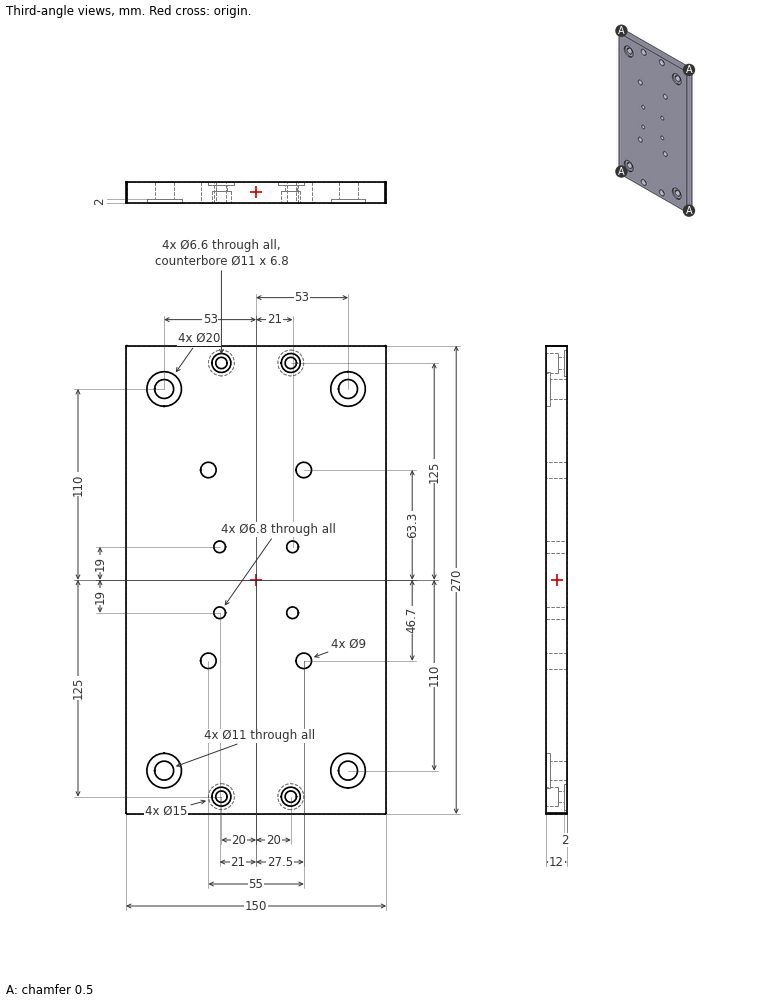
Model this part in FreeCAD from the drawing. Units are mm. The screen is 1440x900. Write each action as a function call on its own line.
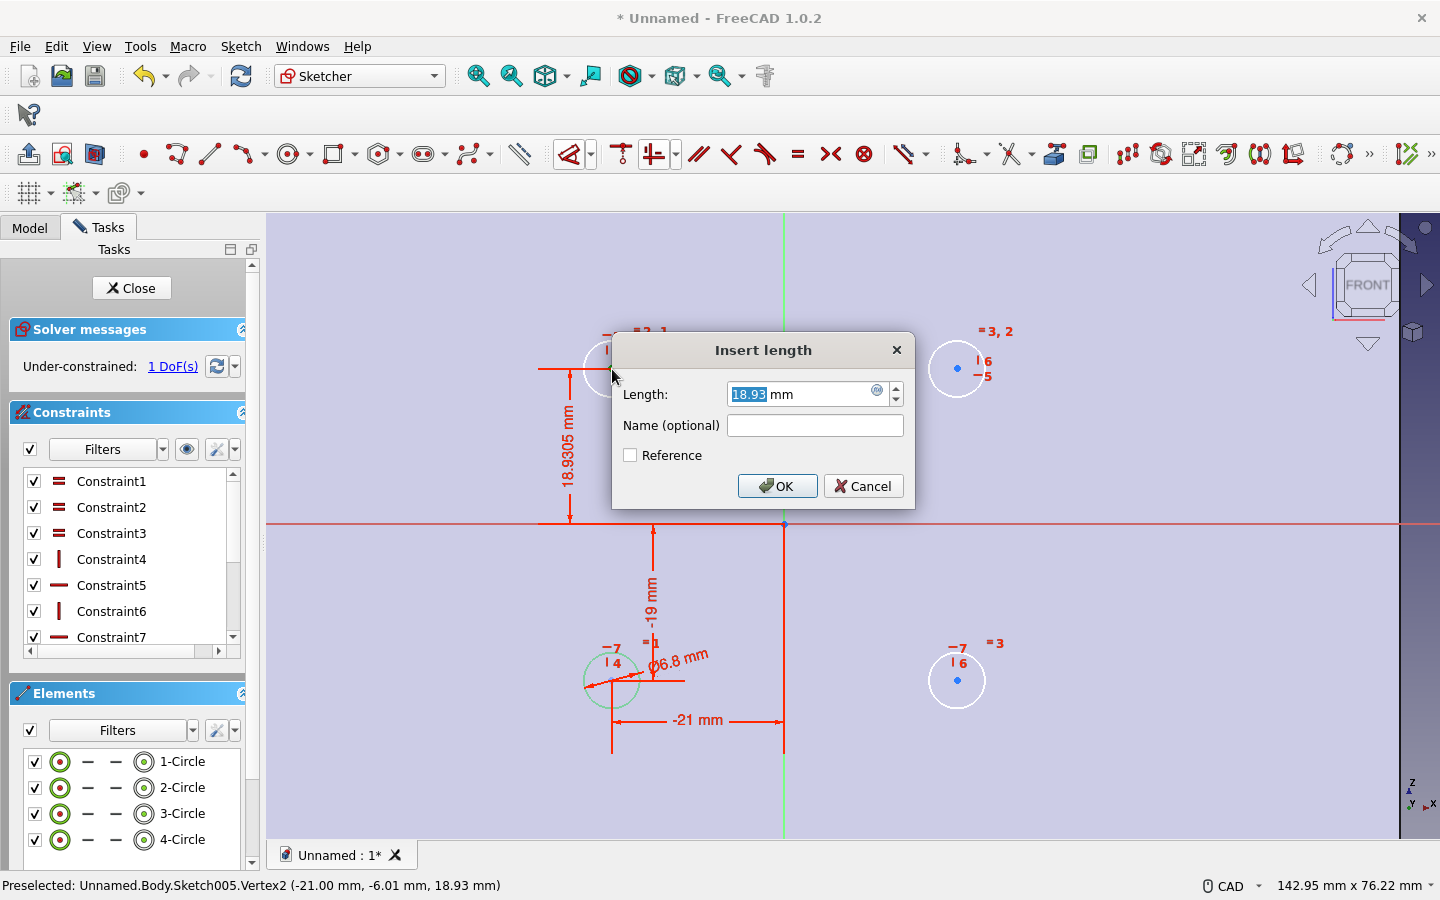
text(19)
key(Return)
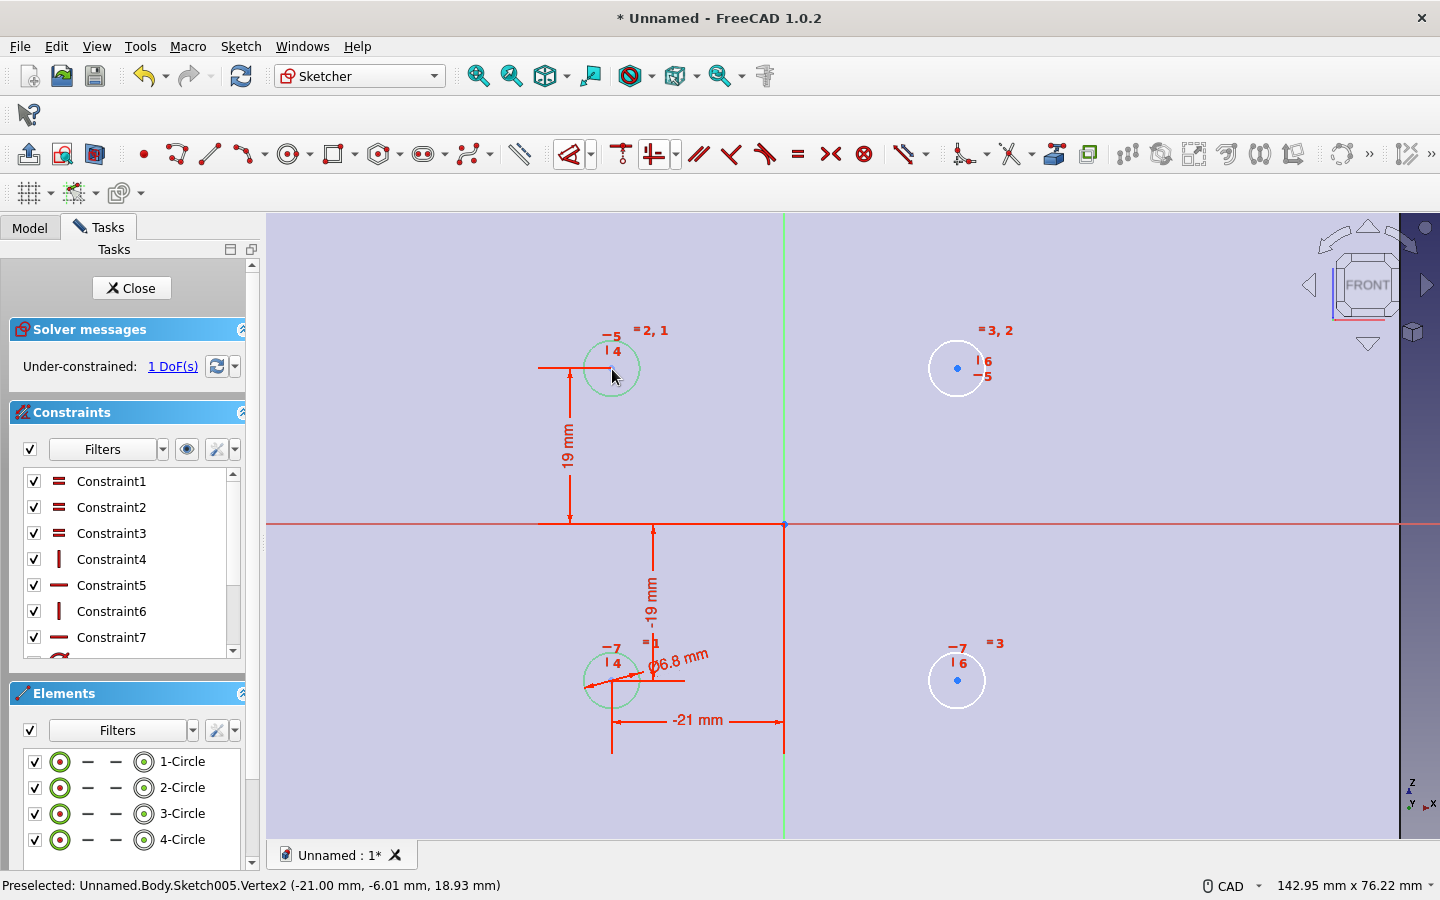
click(957, 368)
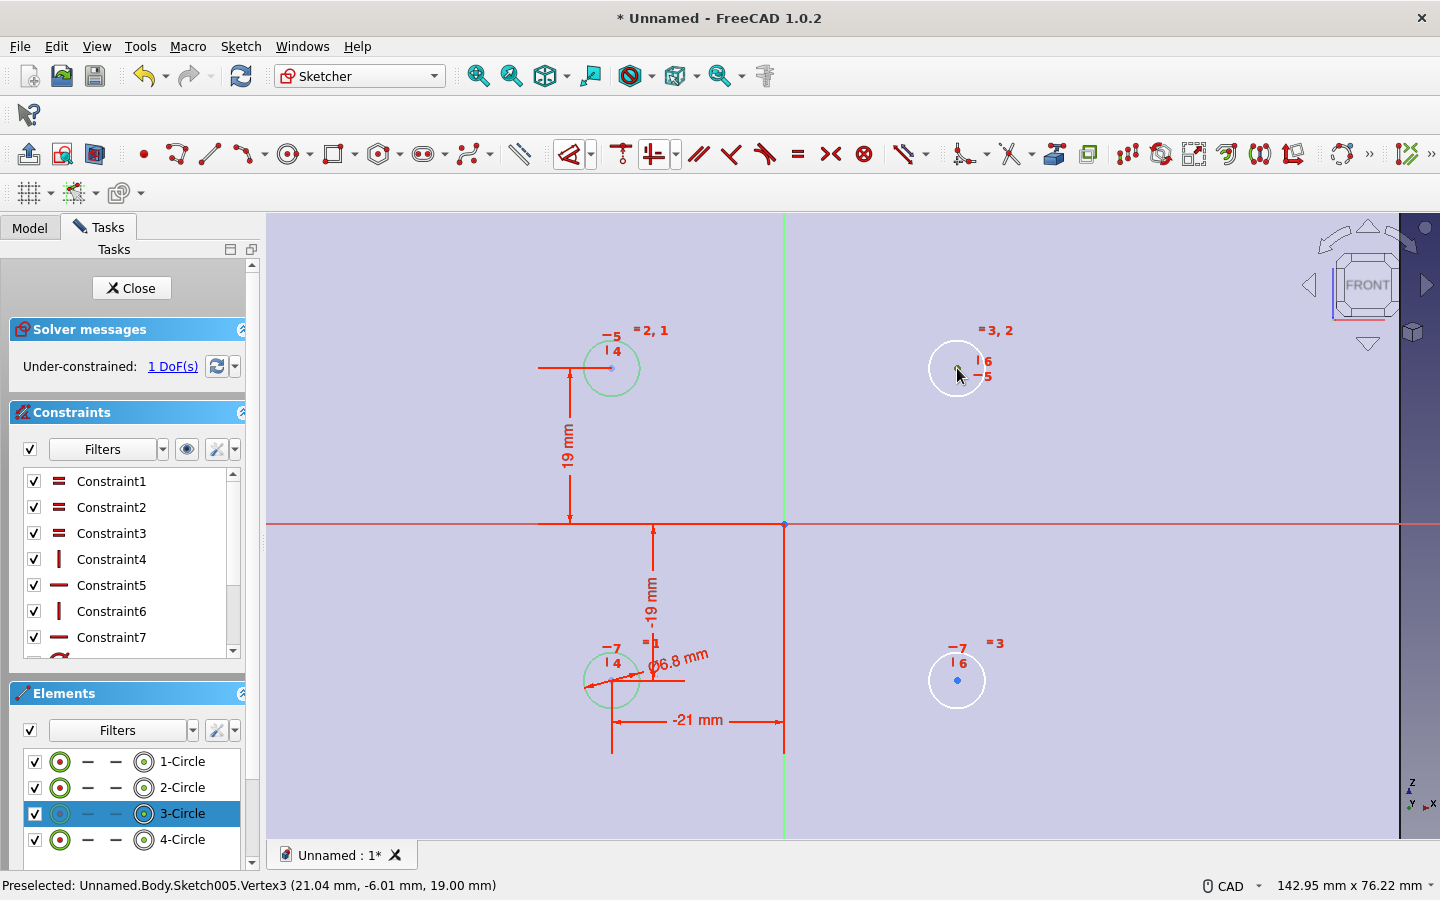
key(l)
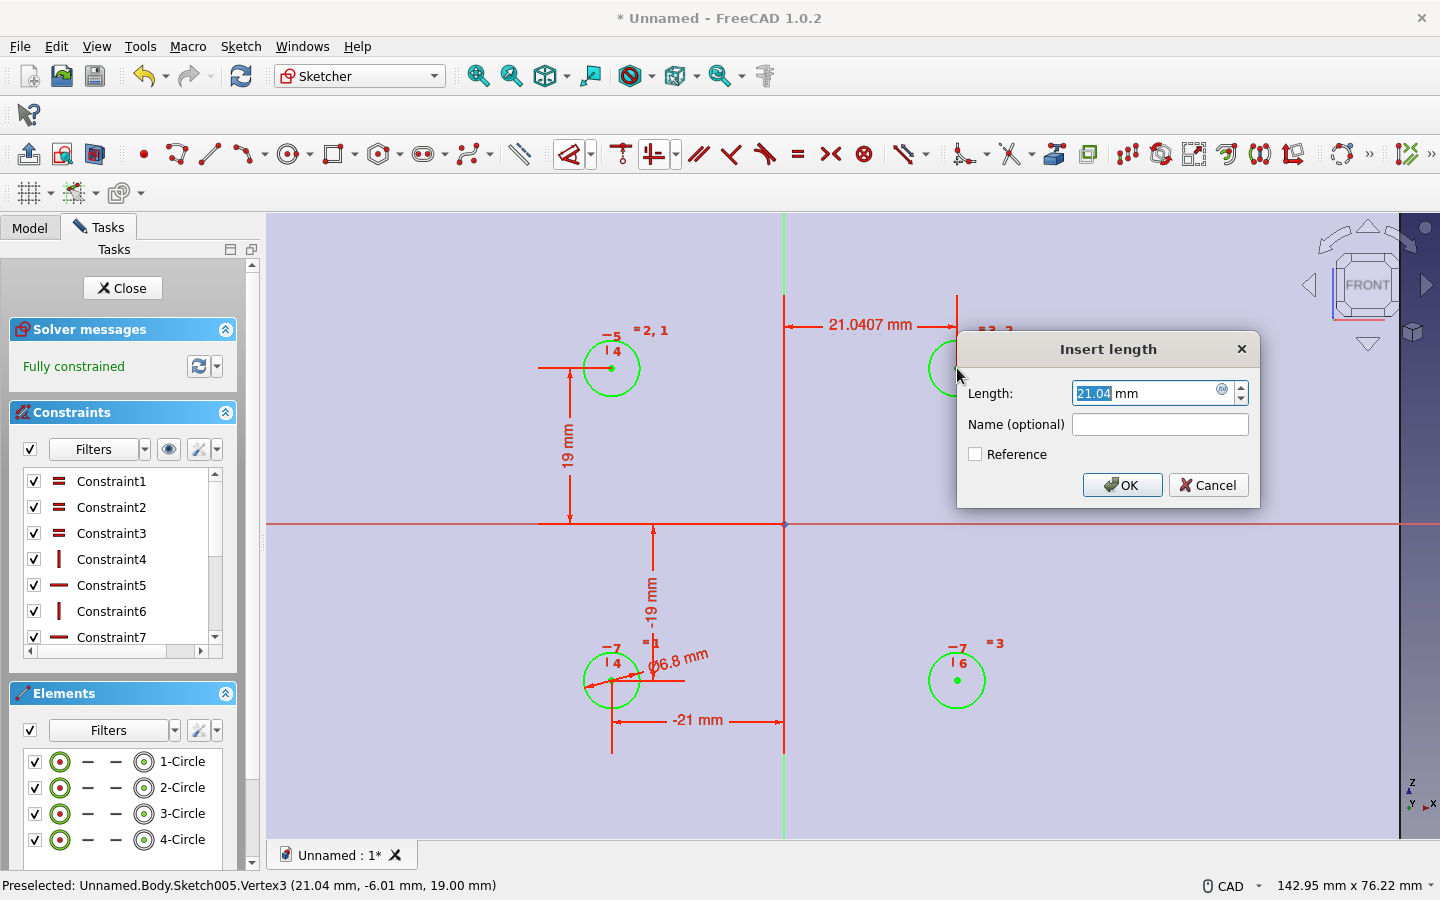
text(21)
key(Return)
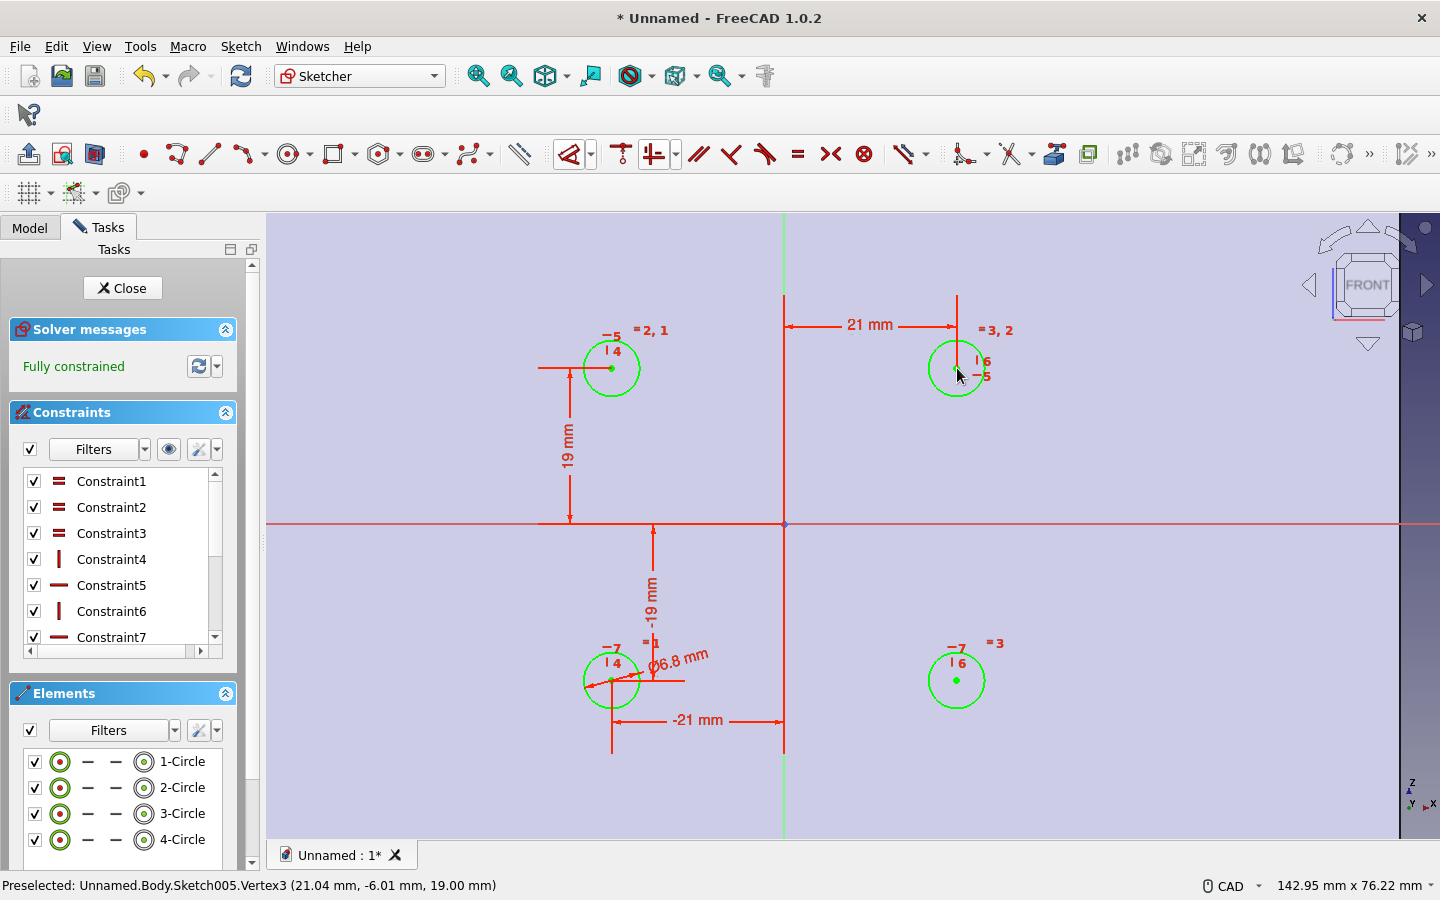
click(123, 288)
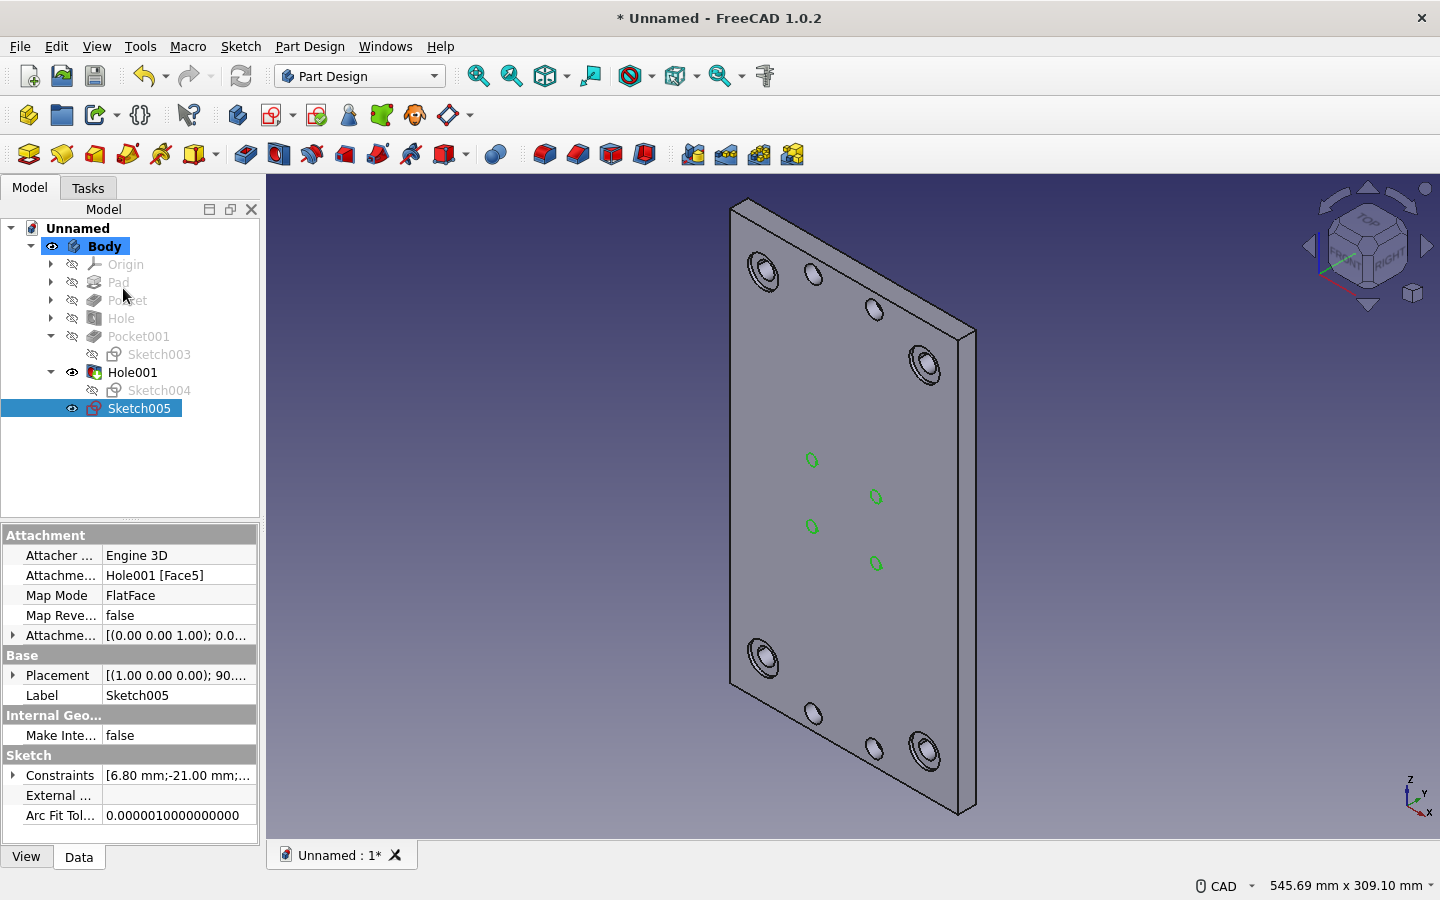
click(279, 154)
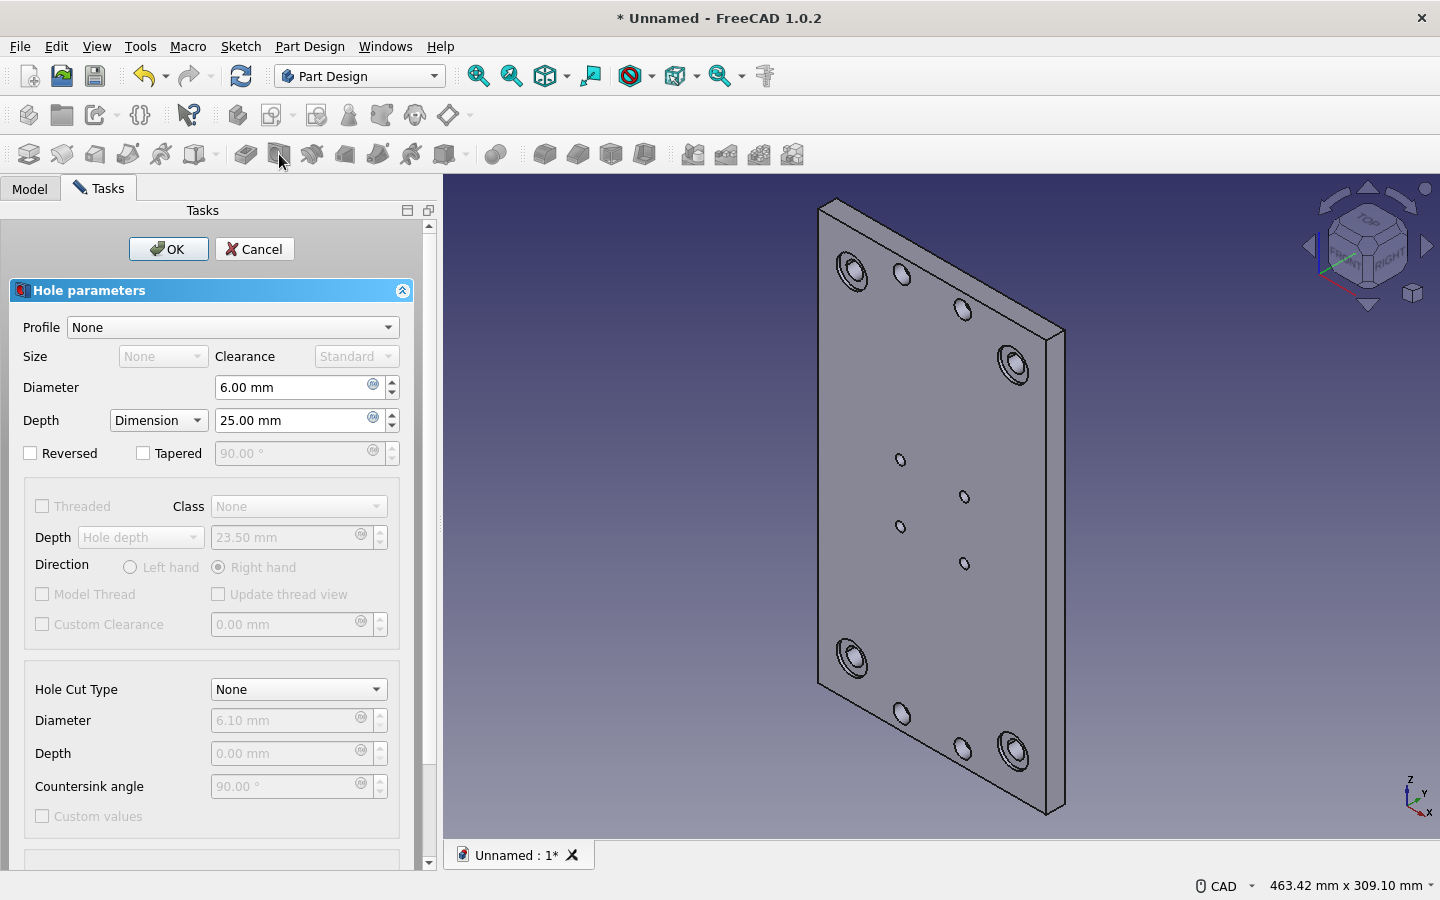
triple_click(300, 388)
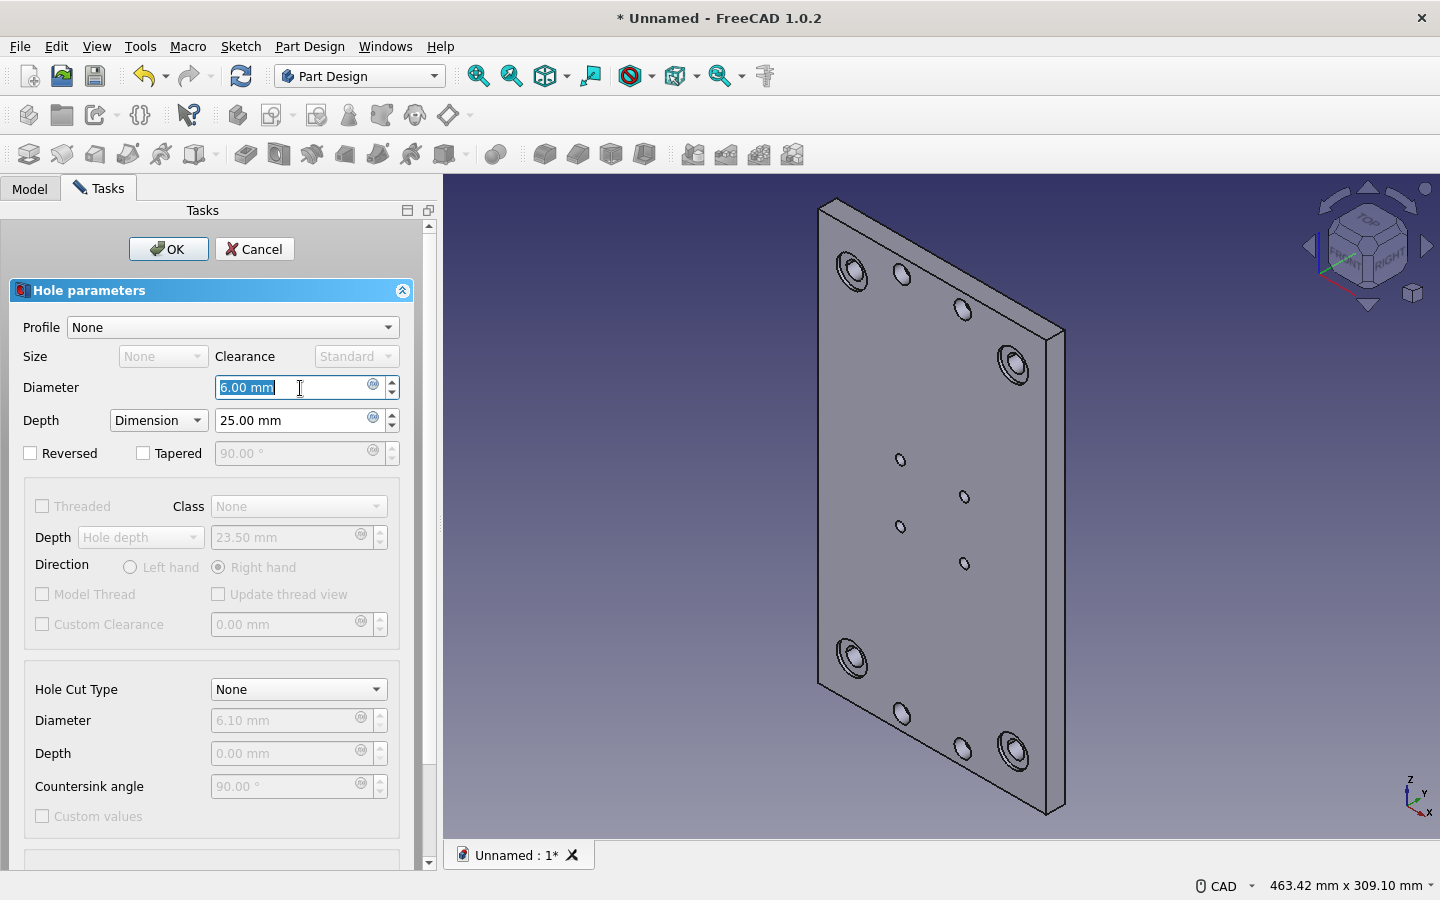
text(6.8)
key(Tab)